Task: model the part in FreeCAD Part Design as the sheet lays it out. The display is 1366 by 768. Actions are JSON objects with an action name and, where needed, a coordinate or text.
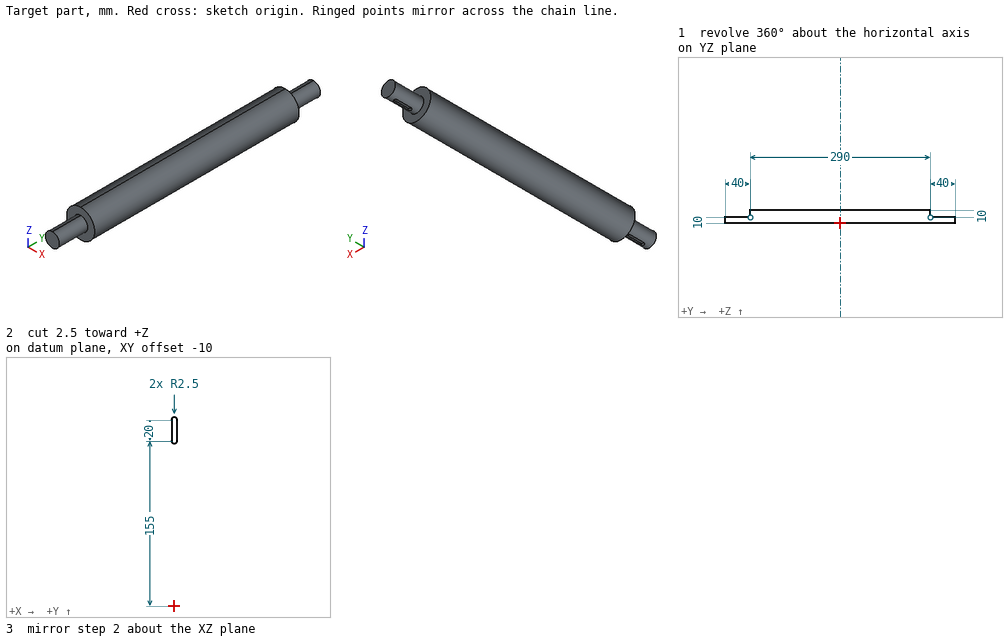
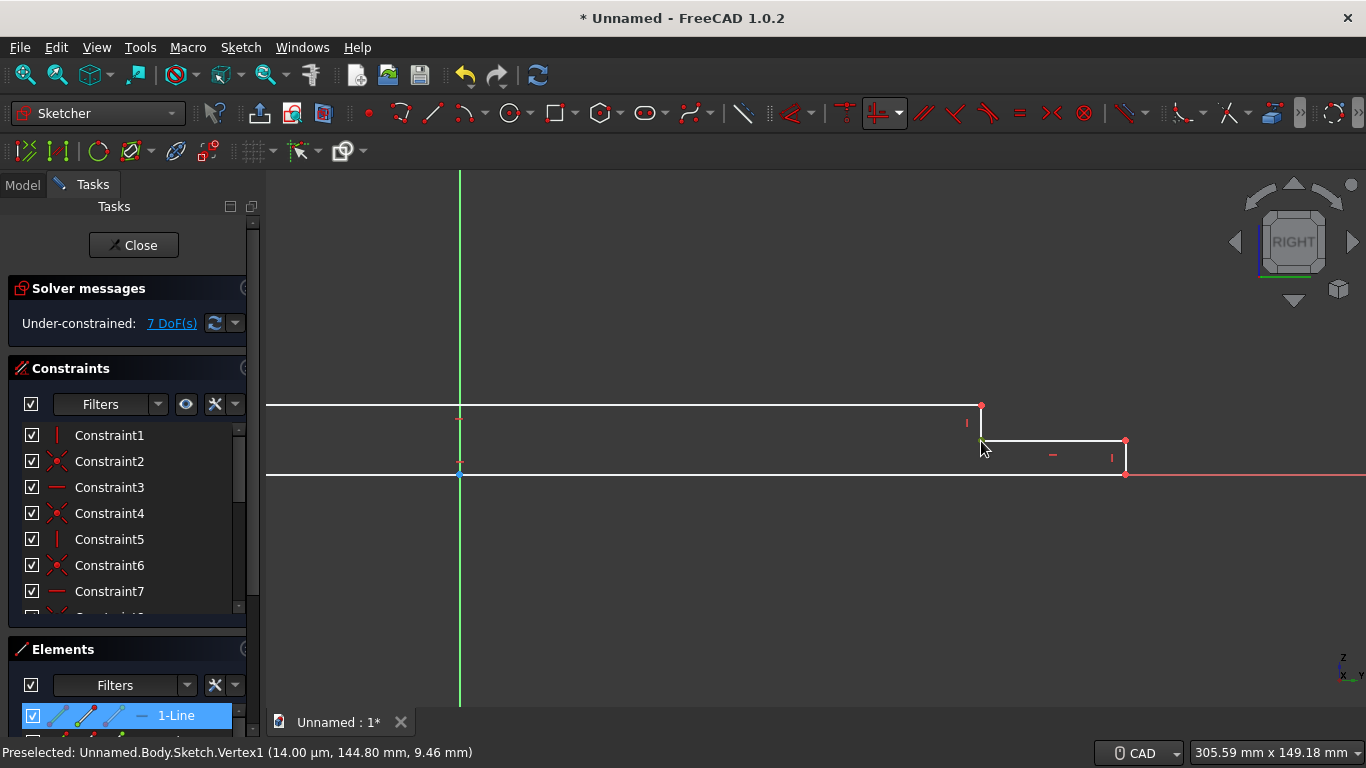
{"action": "scroll", "coordinate": [982, 438], "scroll_direction": "down", "scroll_amount": 4}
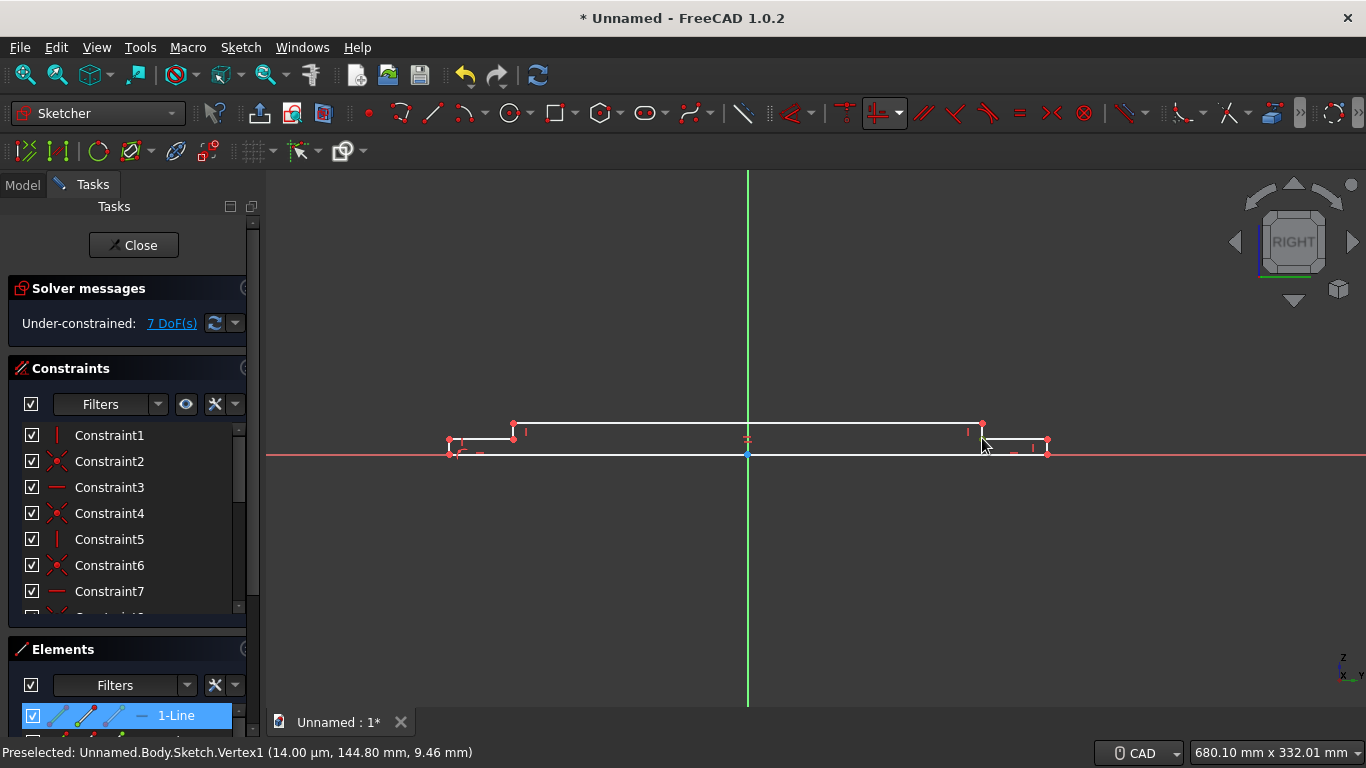
{"action": "left_click", "coordinate": [513, 439]}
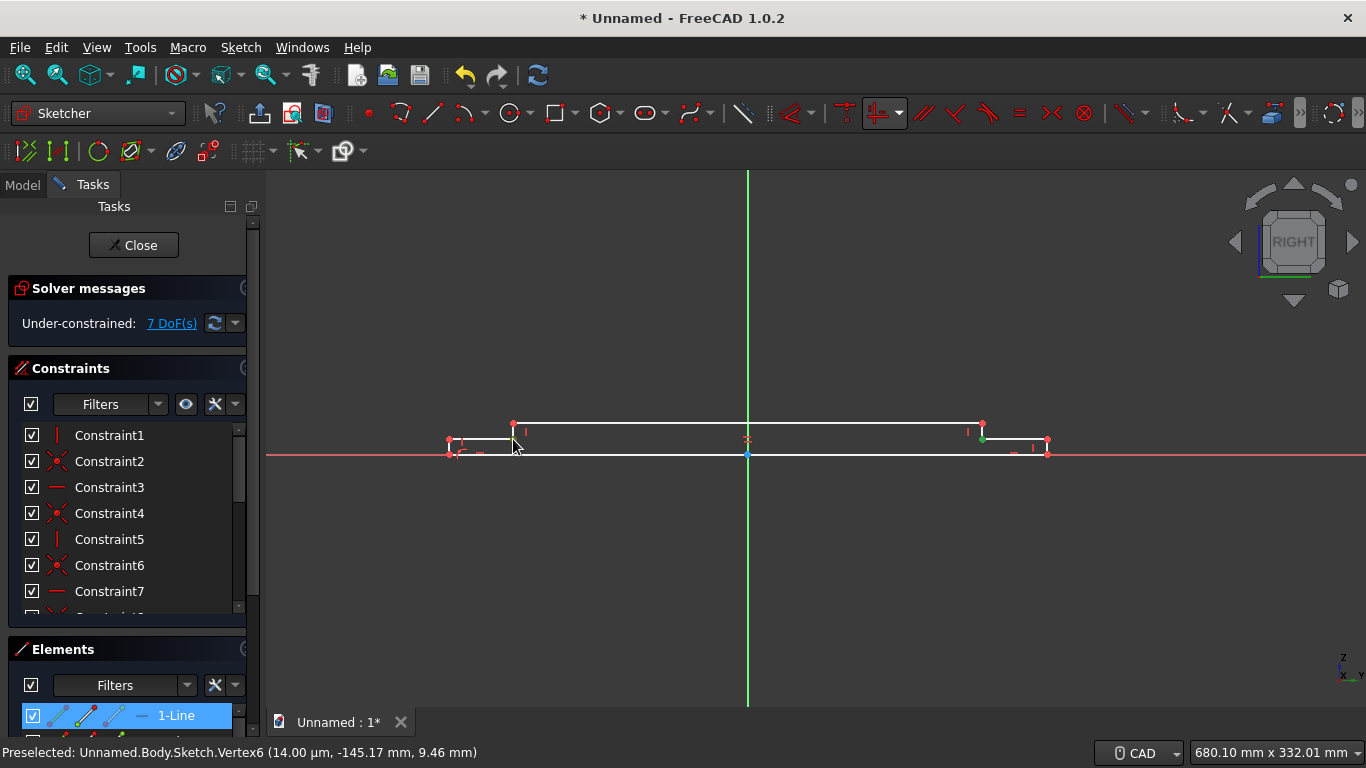
{"action": "left_click", "coordinate": [748, 645]}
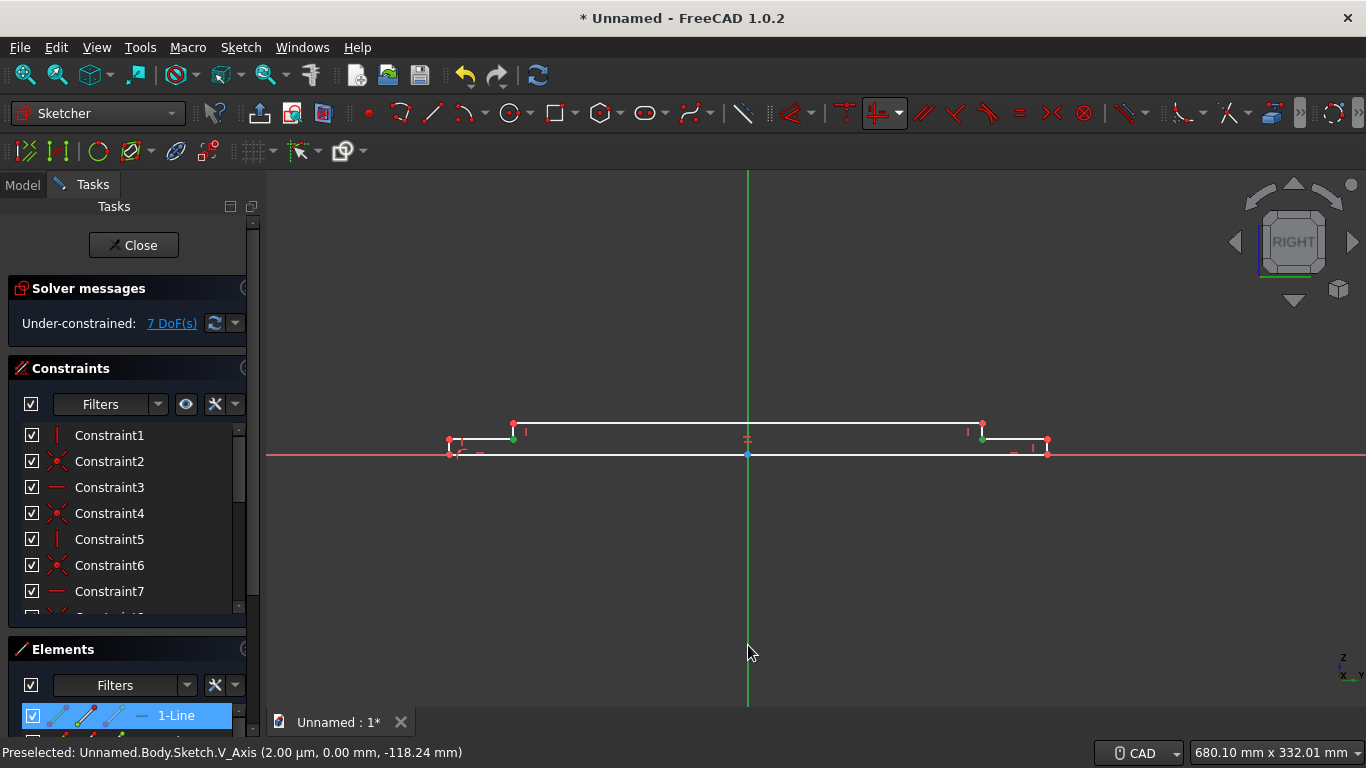
{"action": "key", "text": "s"}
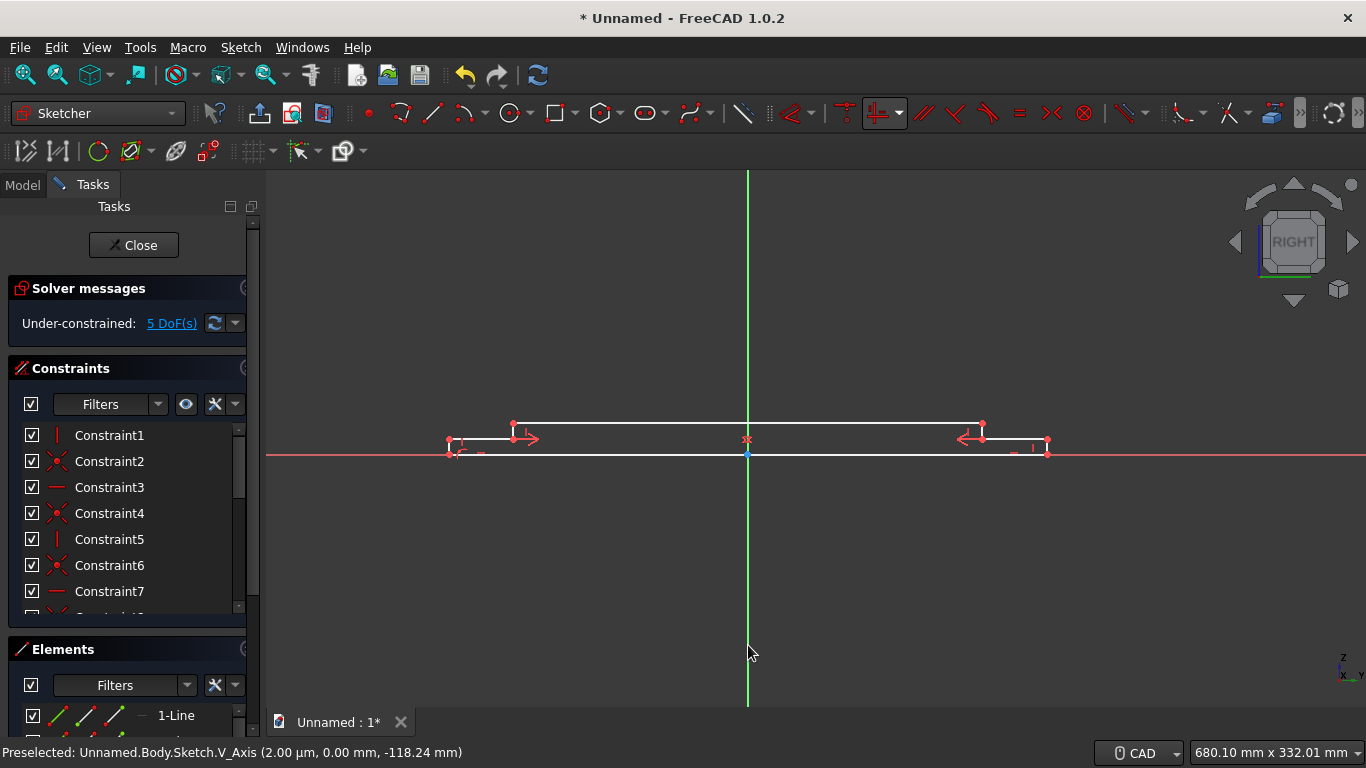
{"action": "key", "text": "d"}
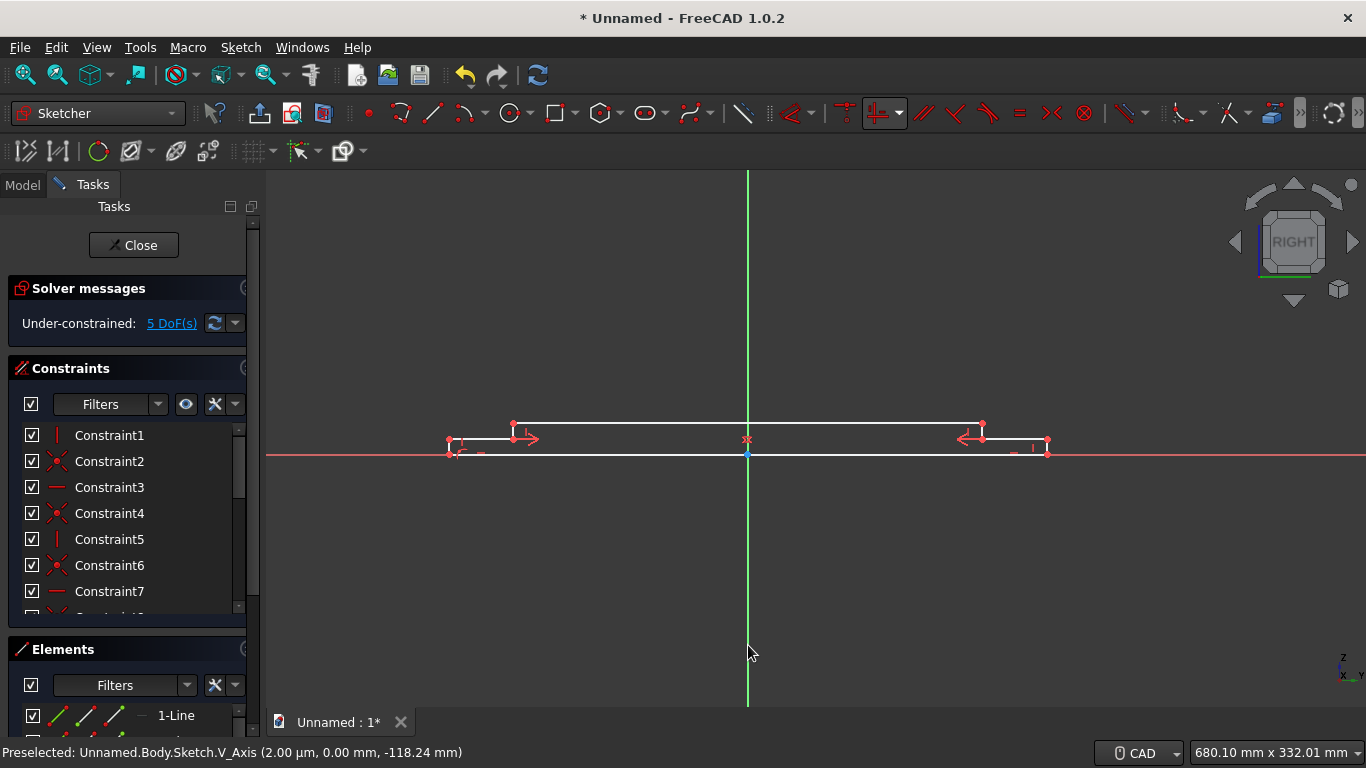
{"action": "scroll", "coordinate": [982, 431], "scroll_direction": "up", "scroll_amount": 5}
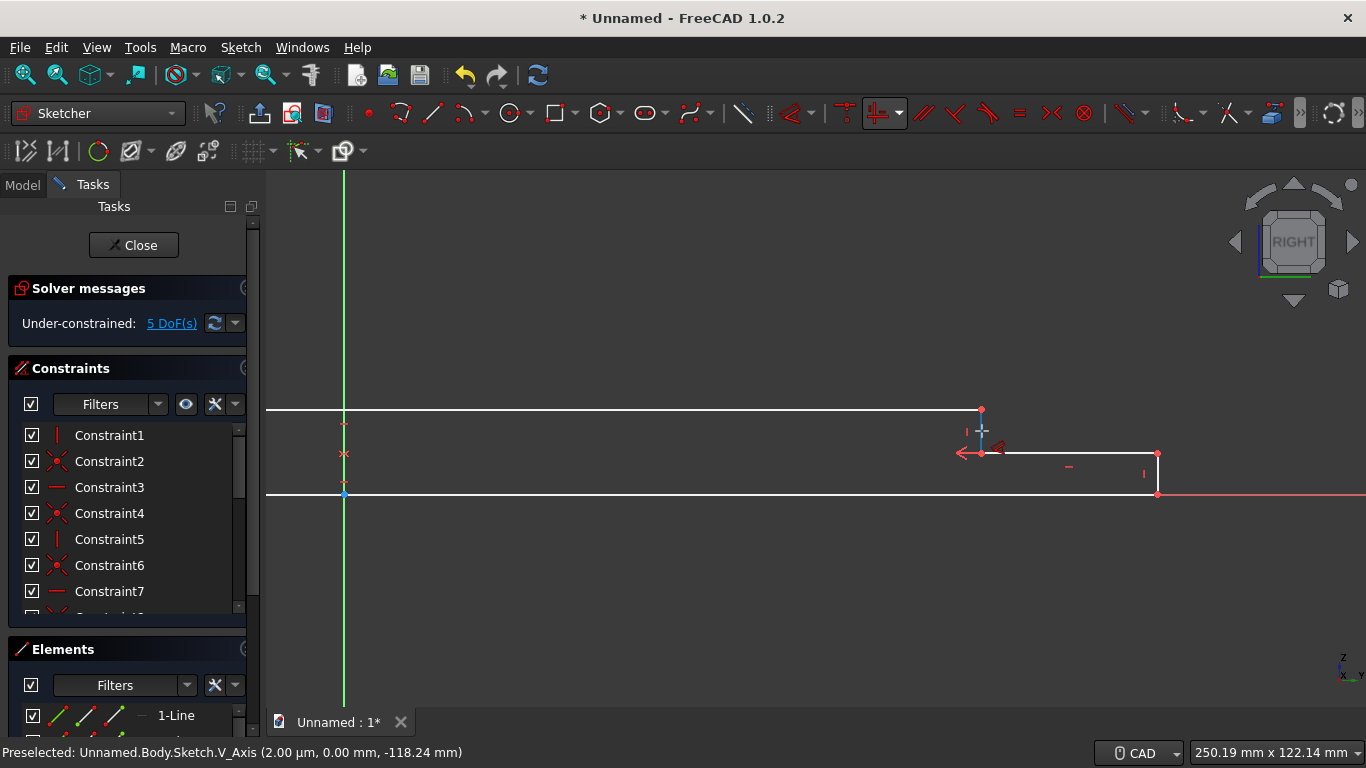
{"action": "left_click", "coordinate": [981, 431]}
{"action": "left_click", "coordinate": [1015, 431]}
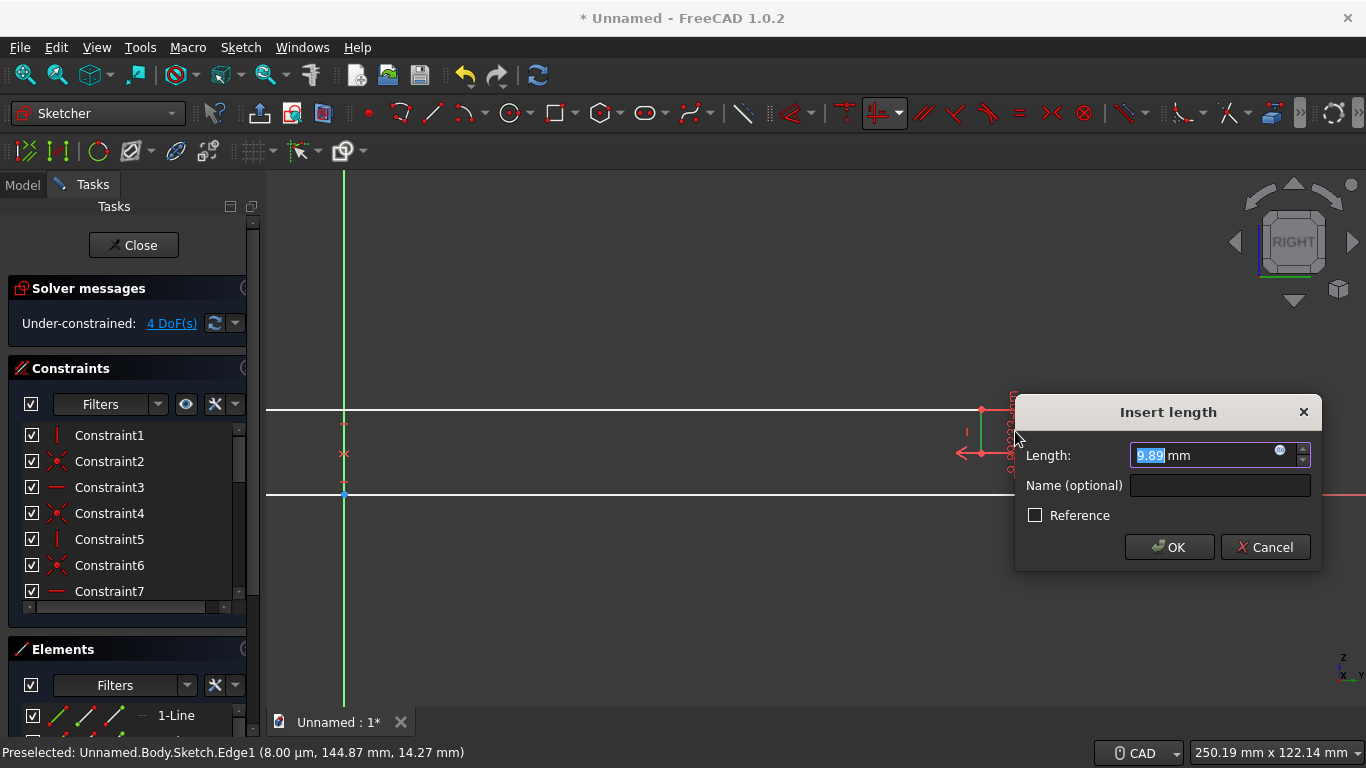
{"action": "type", "text": "10"}
{"action": "key", "text": "Return"}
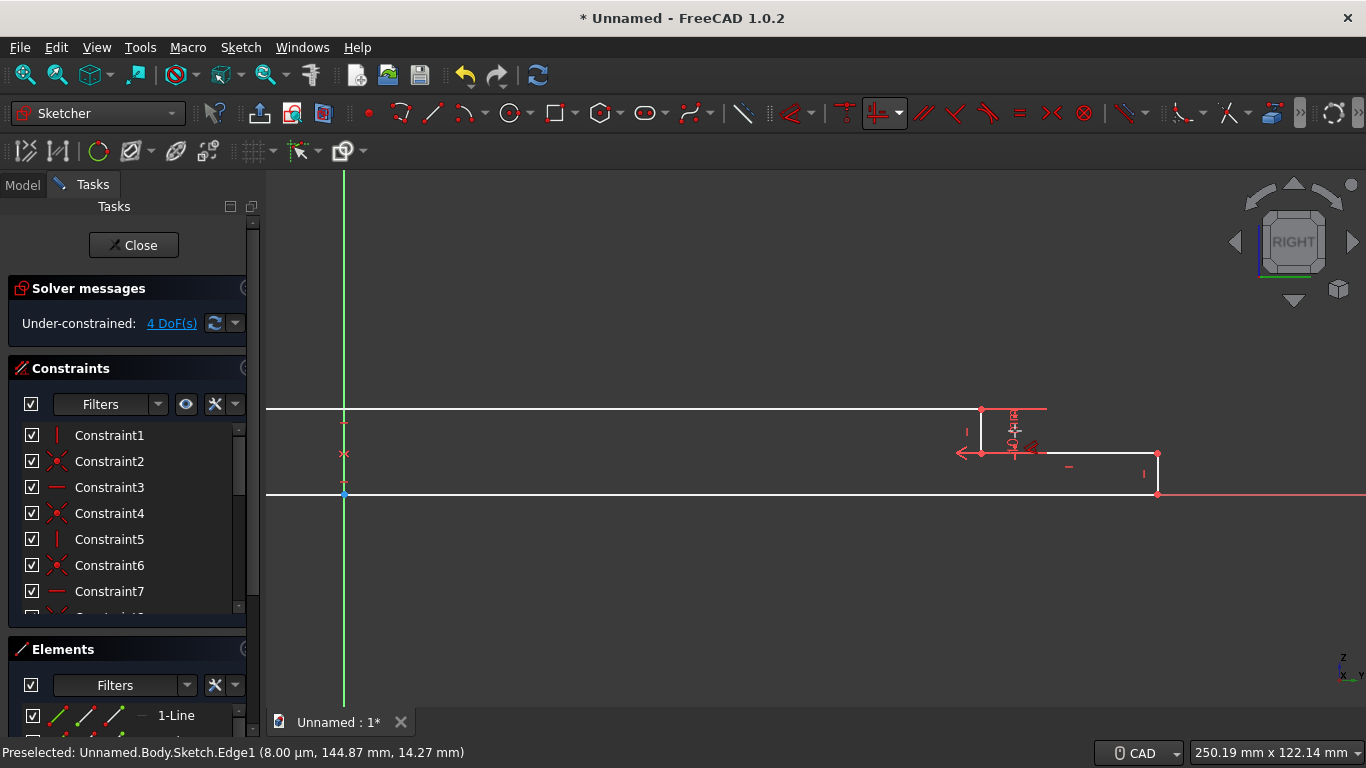
{"action": "scroll", "coordinate": [982, 431], "scroll_direction": "down", "scroll_amount": 5}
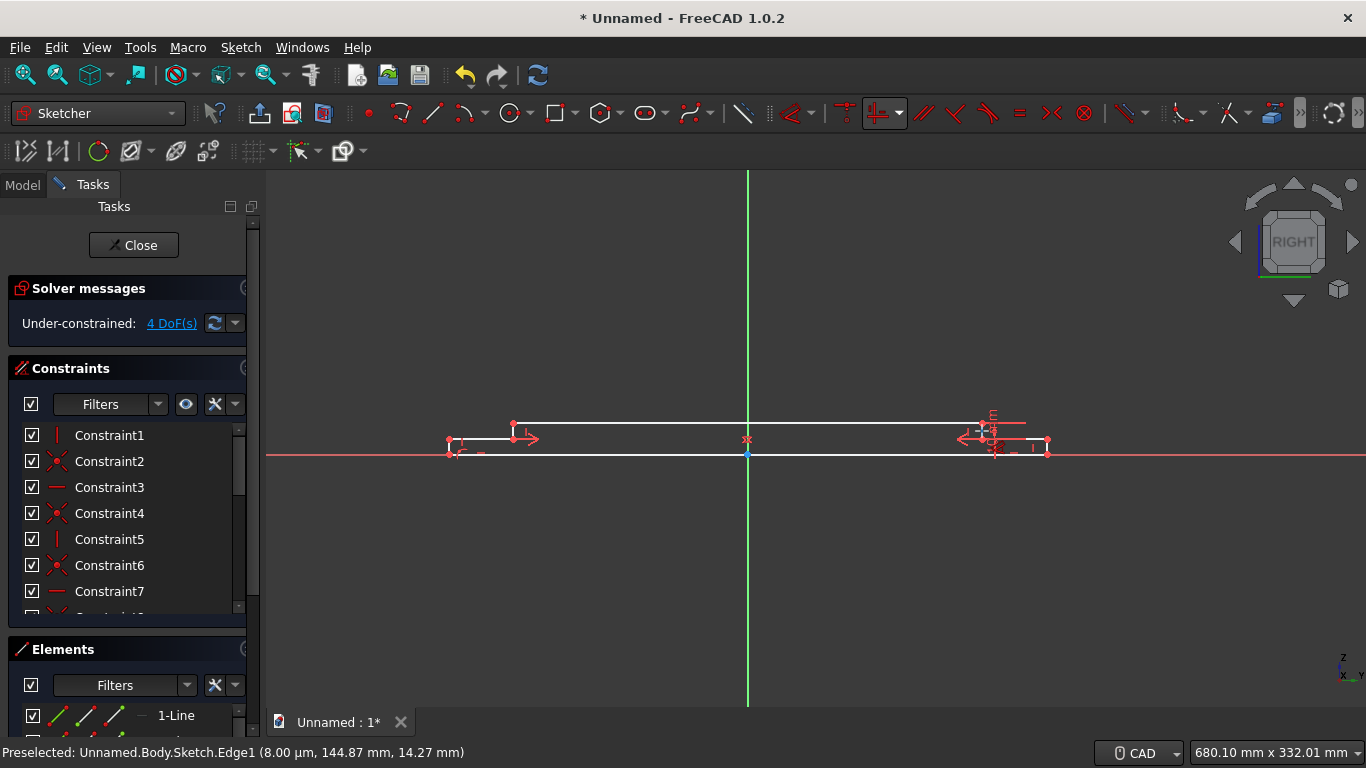
{"action": "left_click", "coordinate": [494, 439]}
{"action": "left_click", "coordinate": [481, 473]}